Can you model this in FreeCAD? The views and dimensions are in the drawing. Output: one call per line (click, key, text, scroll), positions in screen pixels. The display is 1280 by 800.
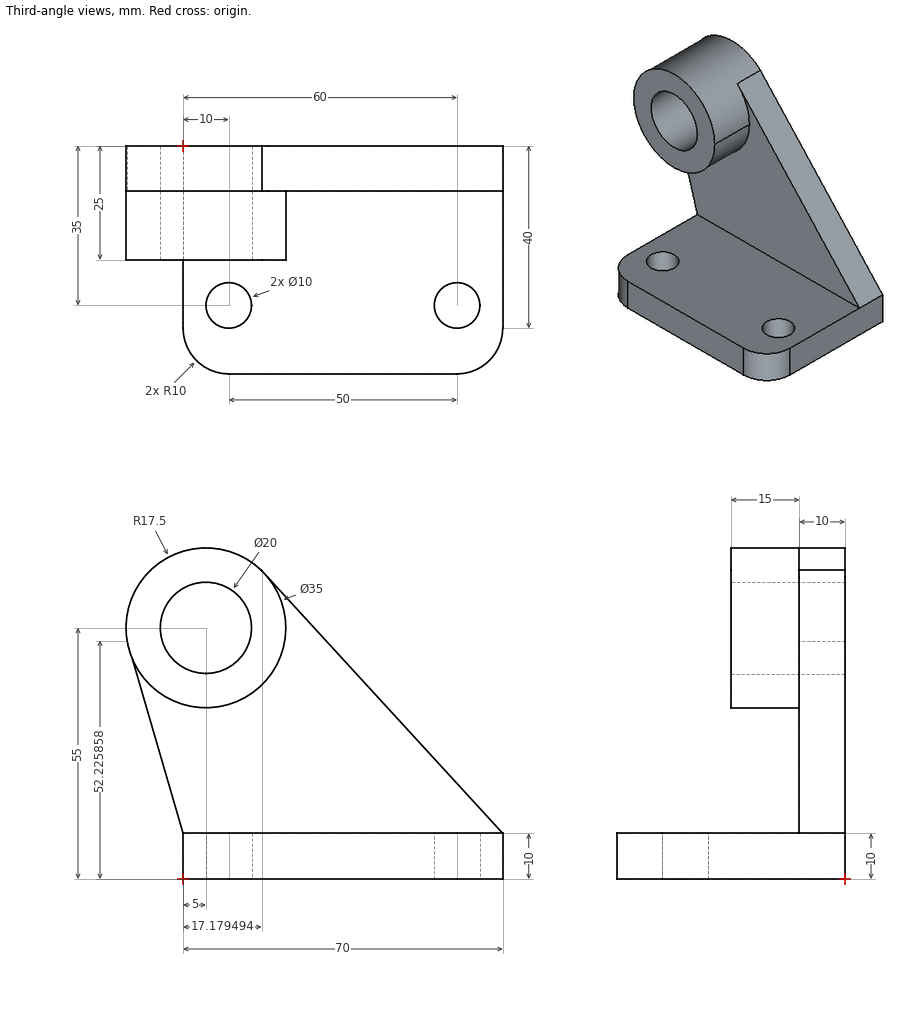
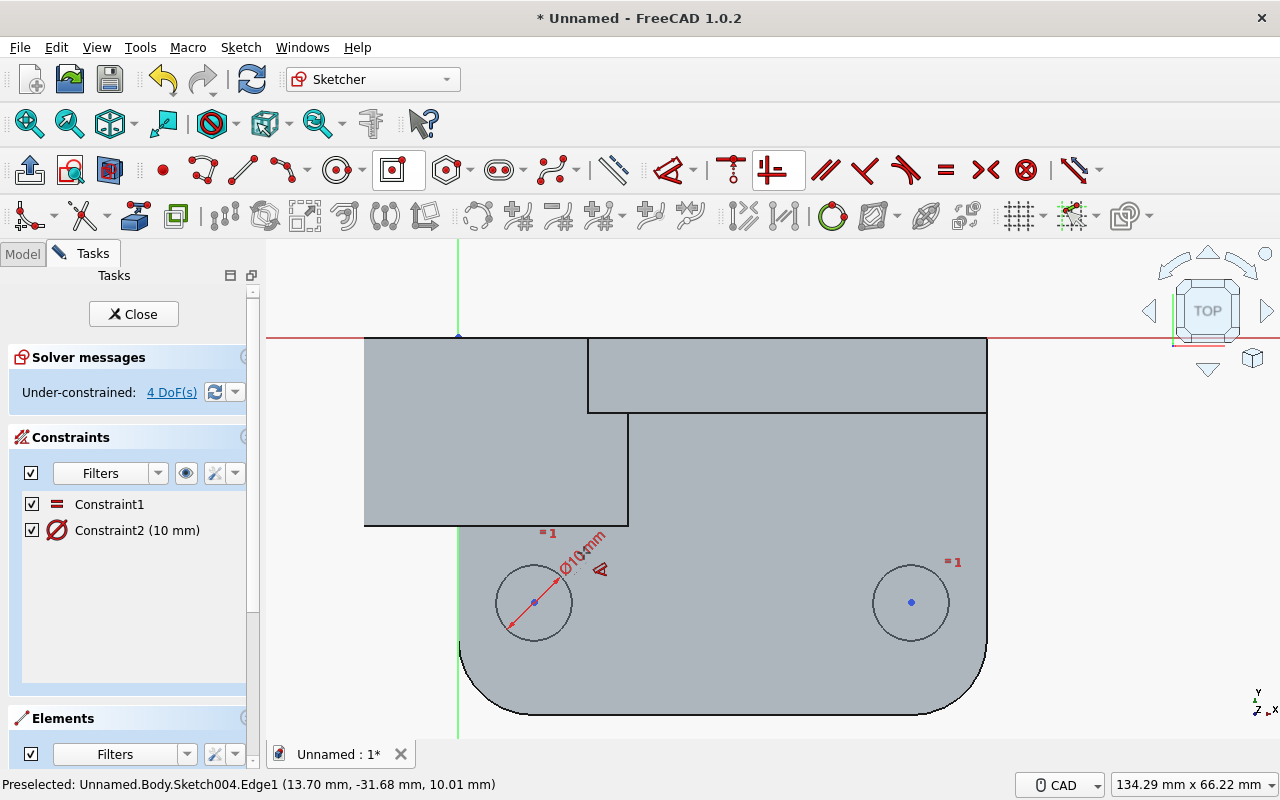
click(534, 603)
click(496, 304)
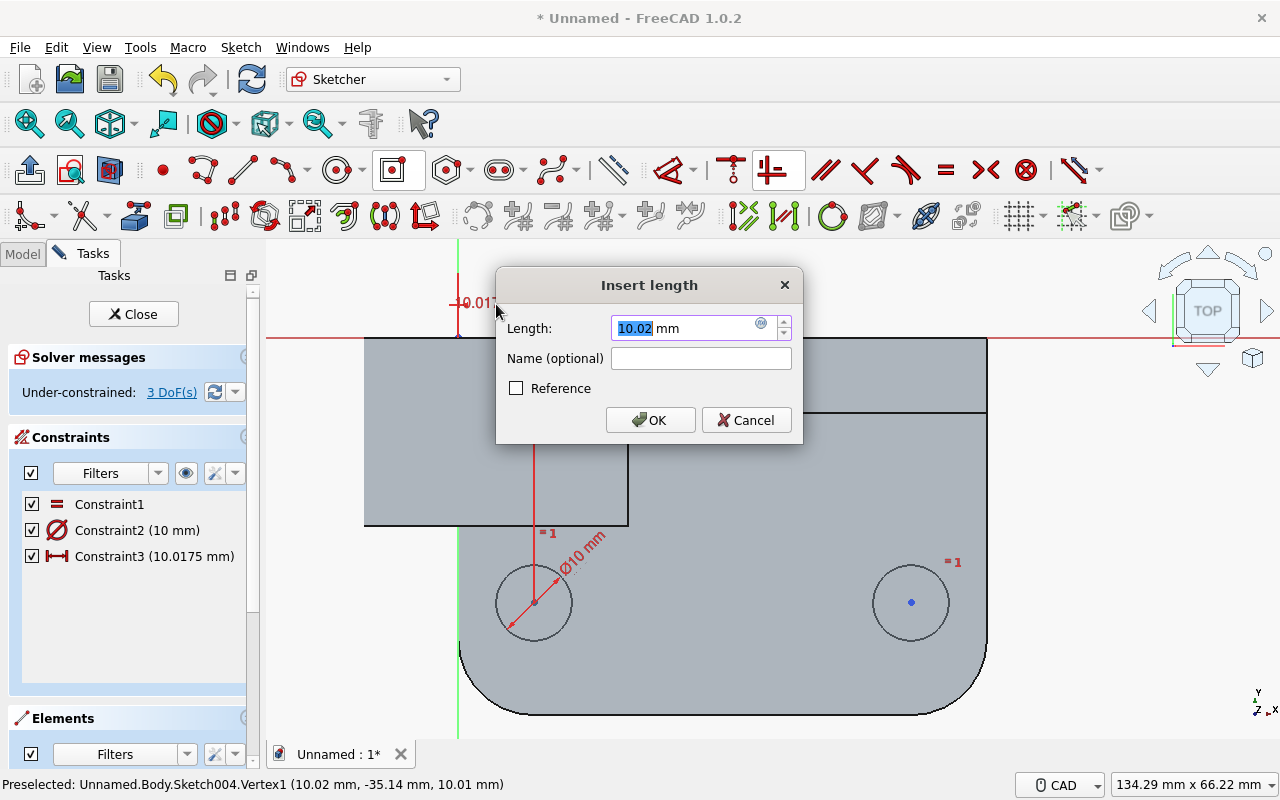
text(10)
key(Return)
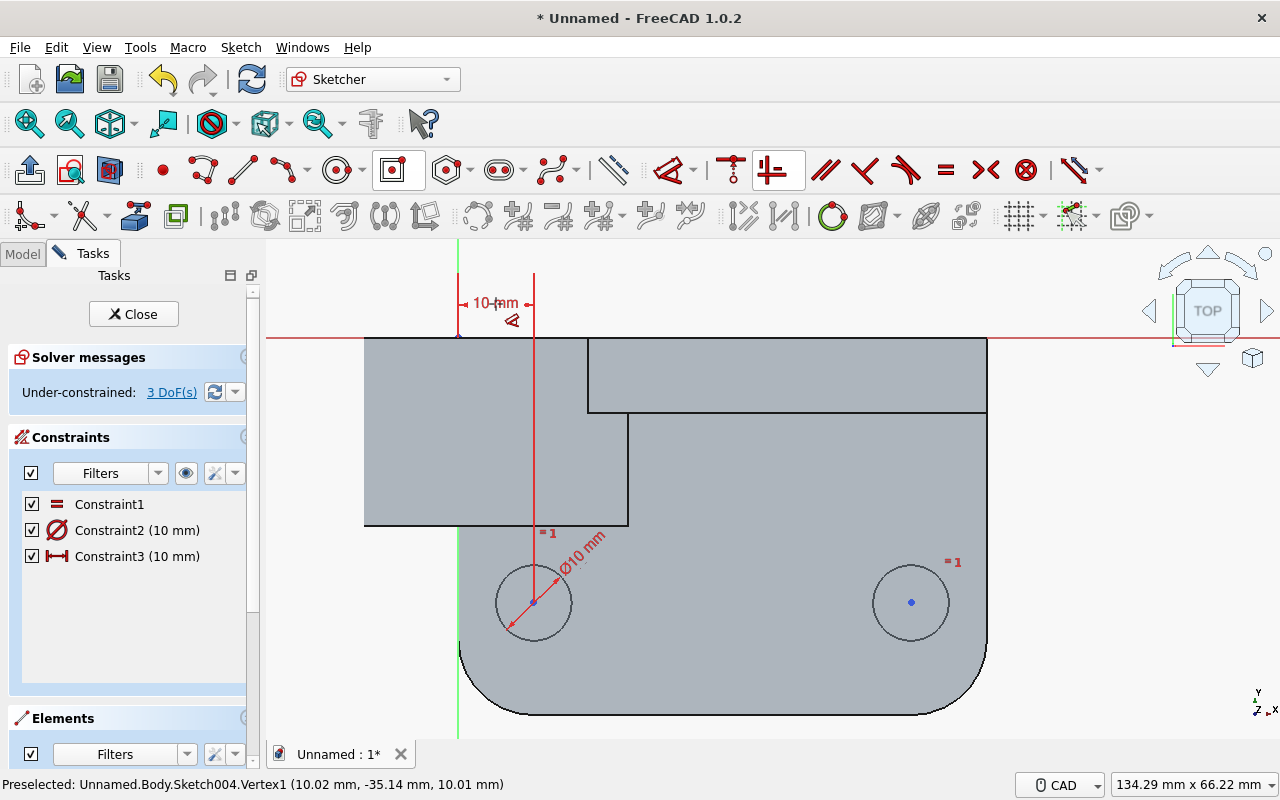
click(534, 603)
click(424, 470)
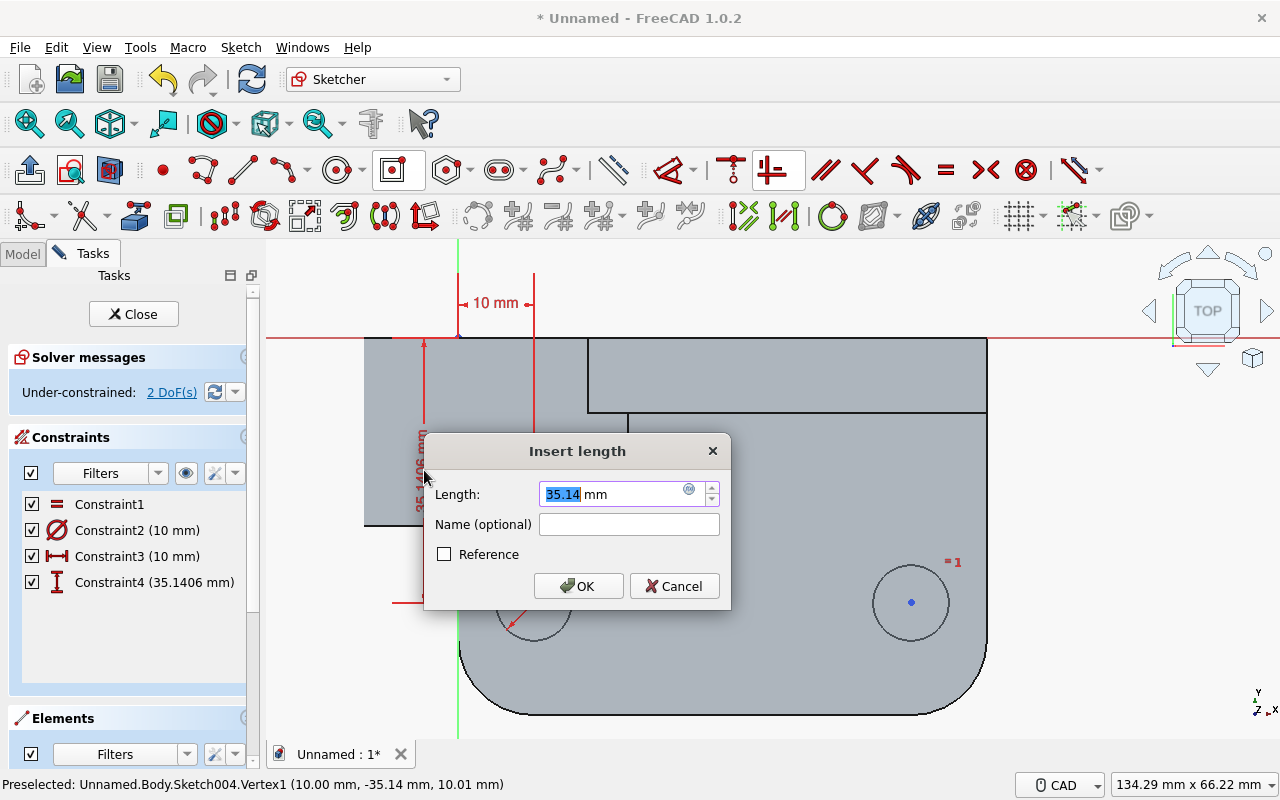
text(35)
key(Return)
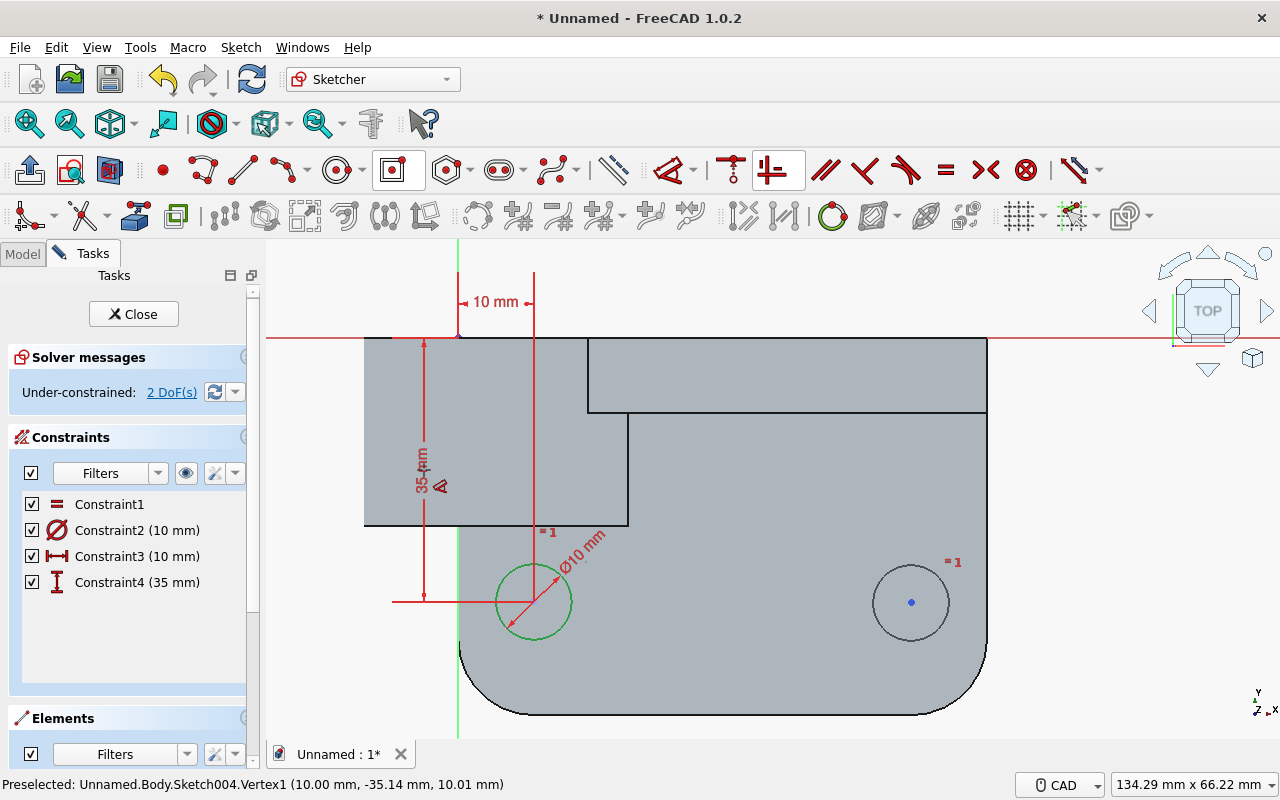
click(911, 603)
click(685, 304)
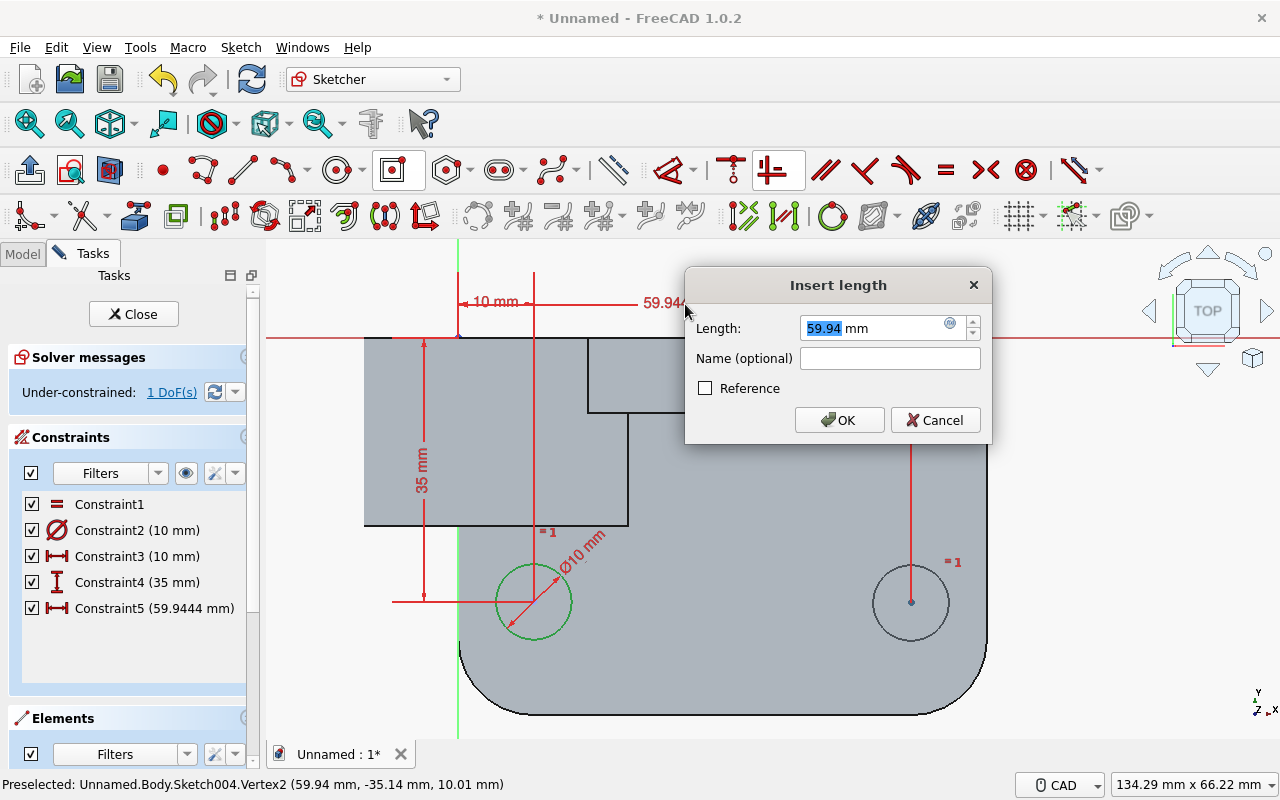
text(60)
key(Return)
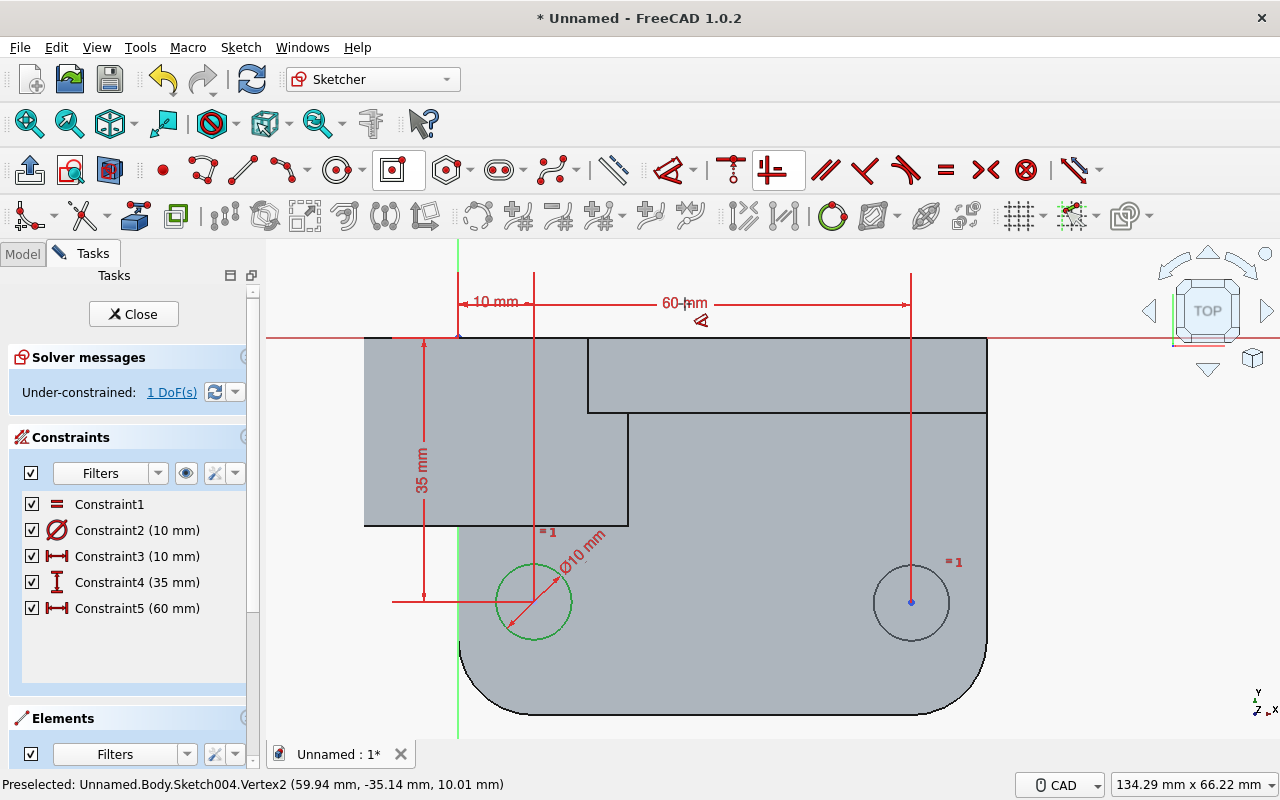
click(911, 603)
click(424, 409)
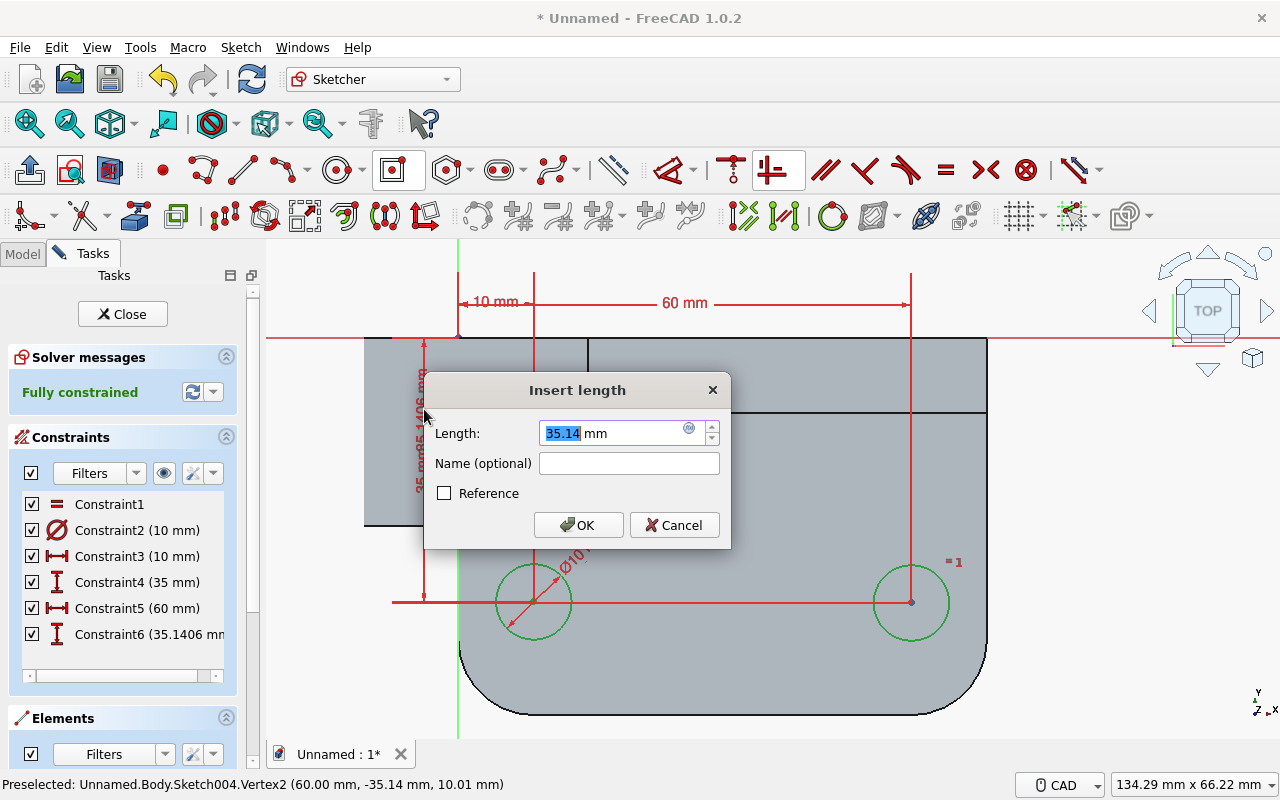
text(35)
key(Return)
key(Escape)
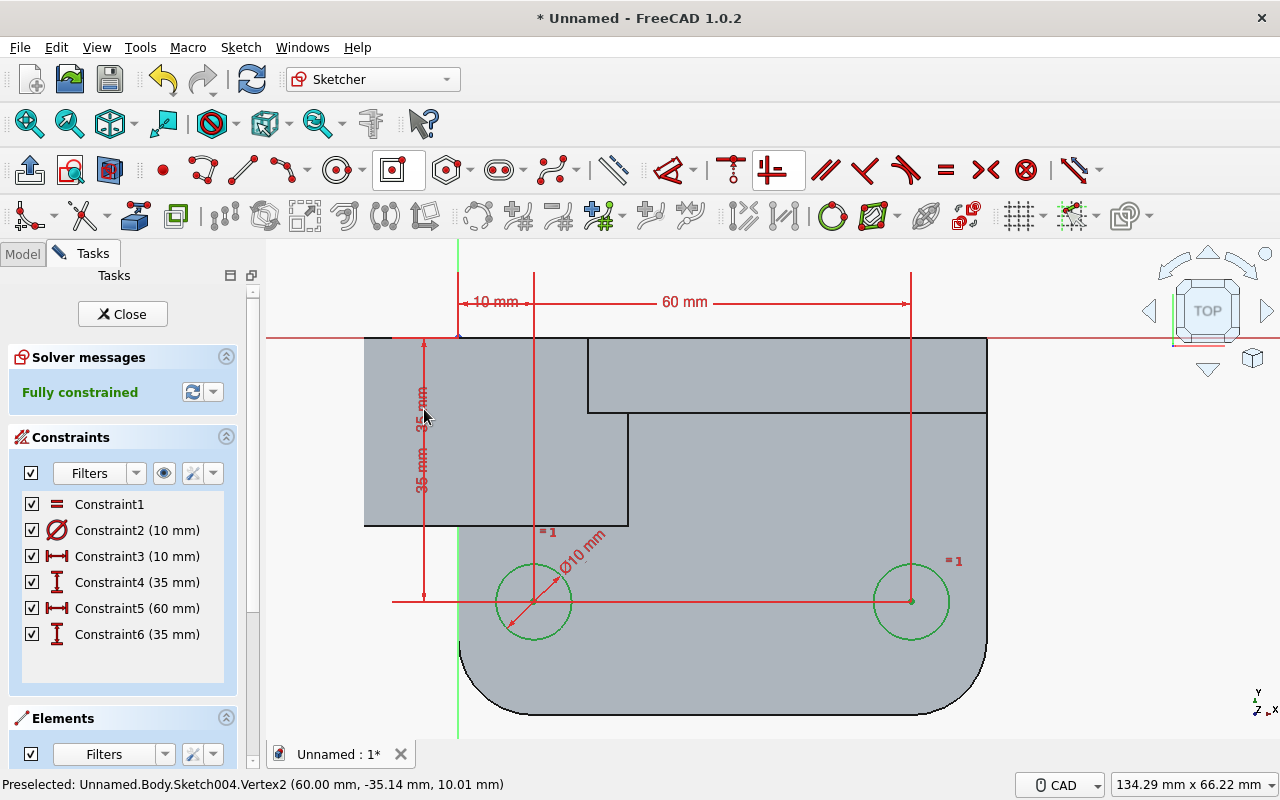
click(123, 314)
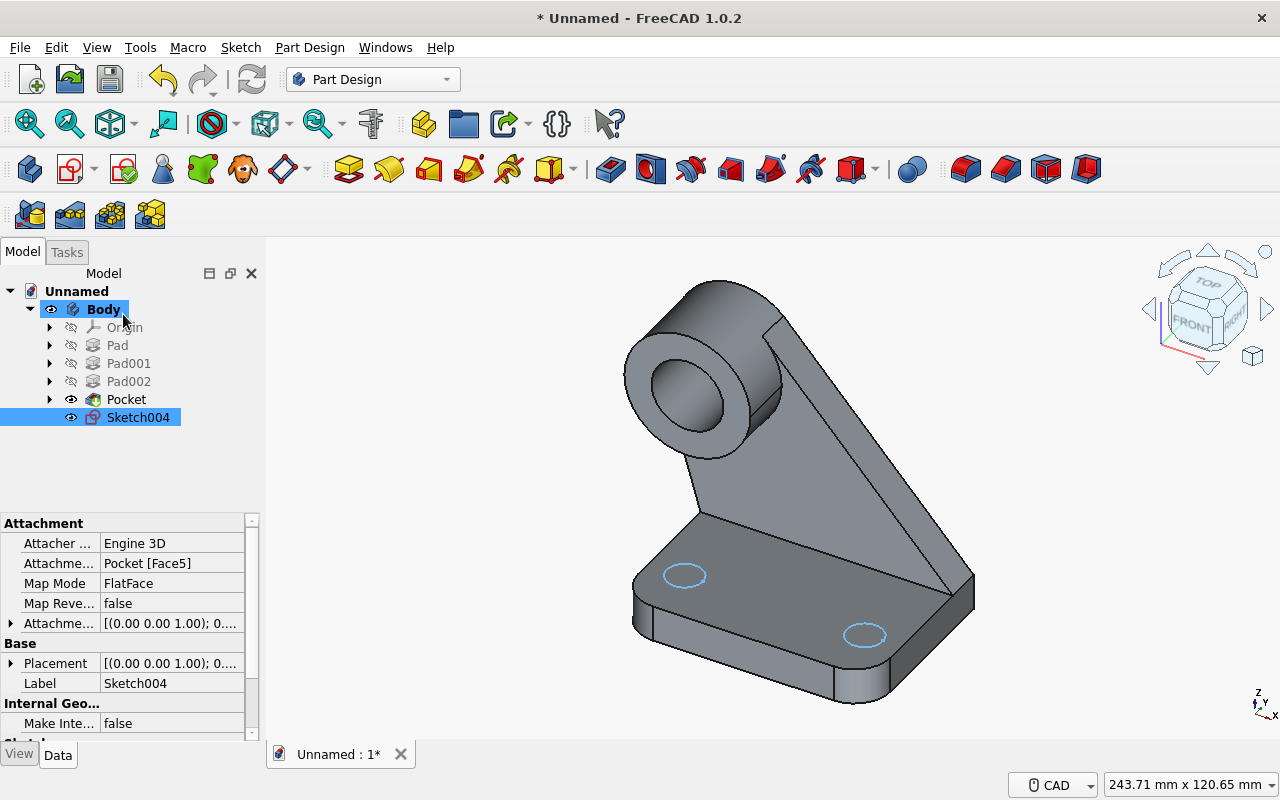
click(612, 170)